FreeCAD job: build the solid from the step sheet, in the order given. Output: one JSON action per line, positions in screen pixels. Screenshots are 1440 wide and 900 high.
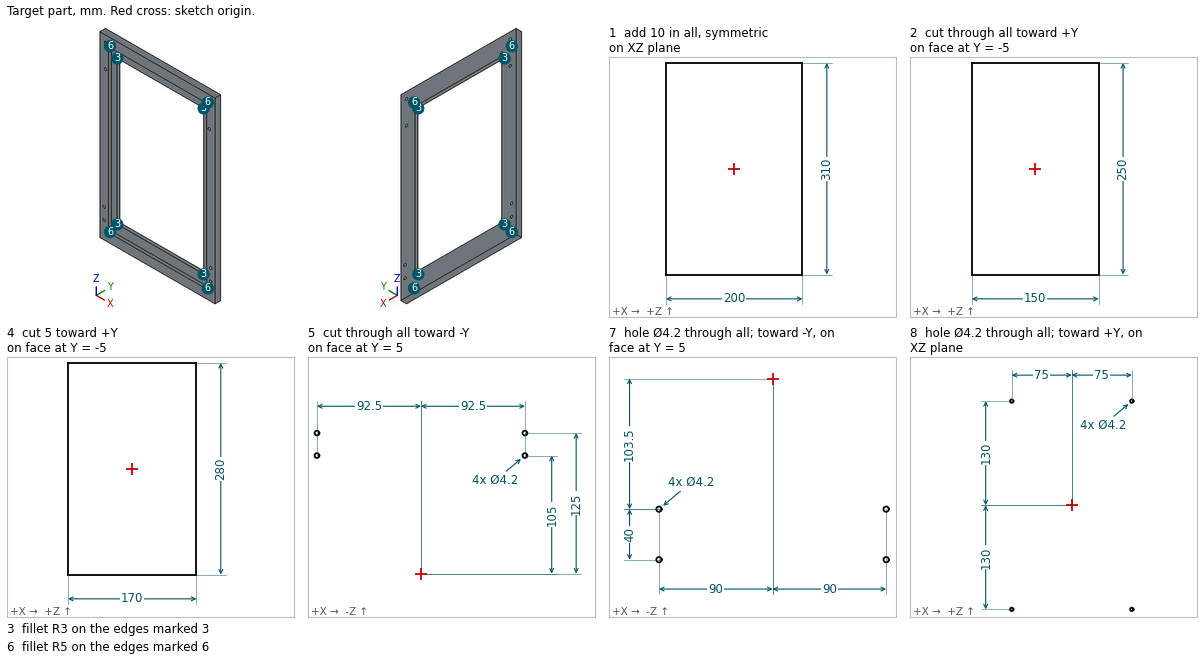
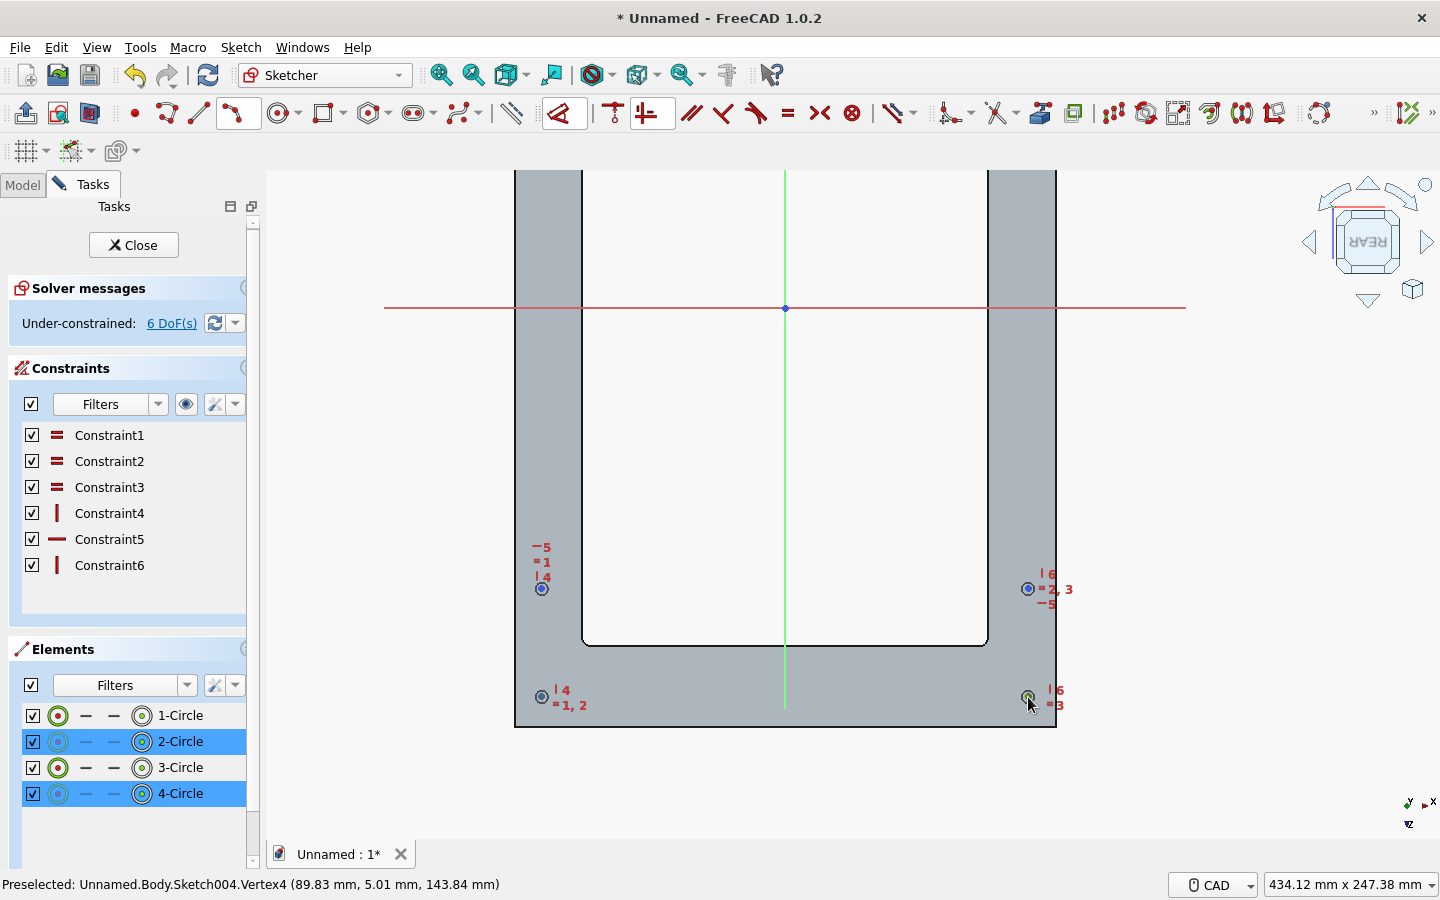
{"action": "left_click", "coordinate": [670, 114]}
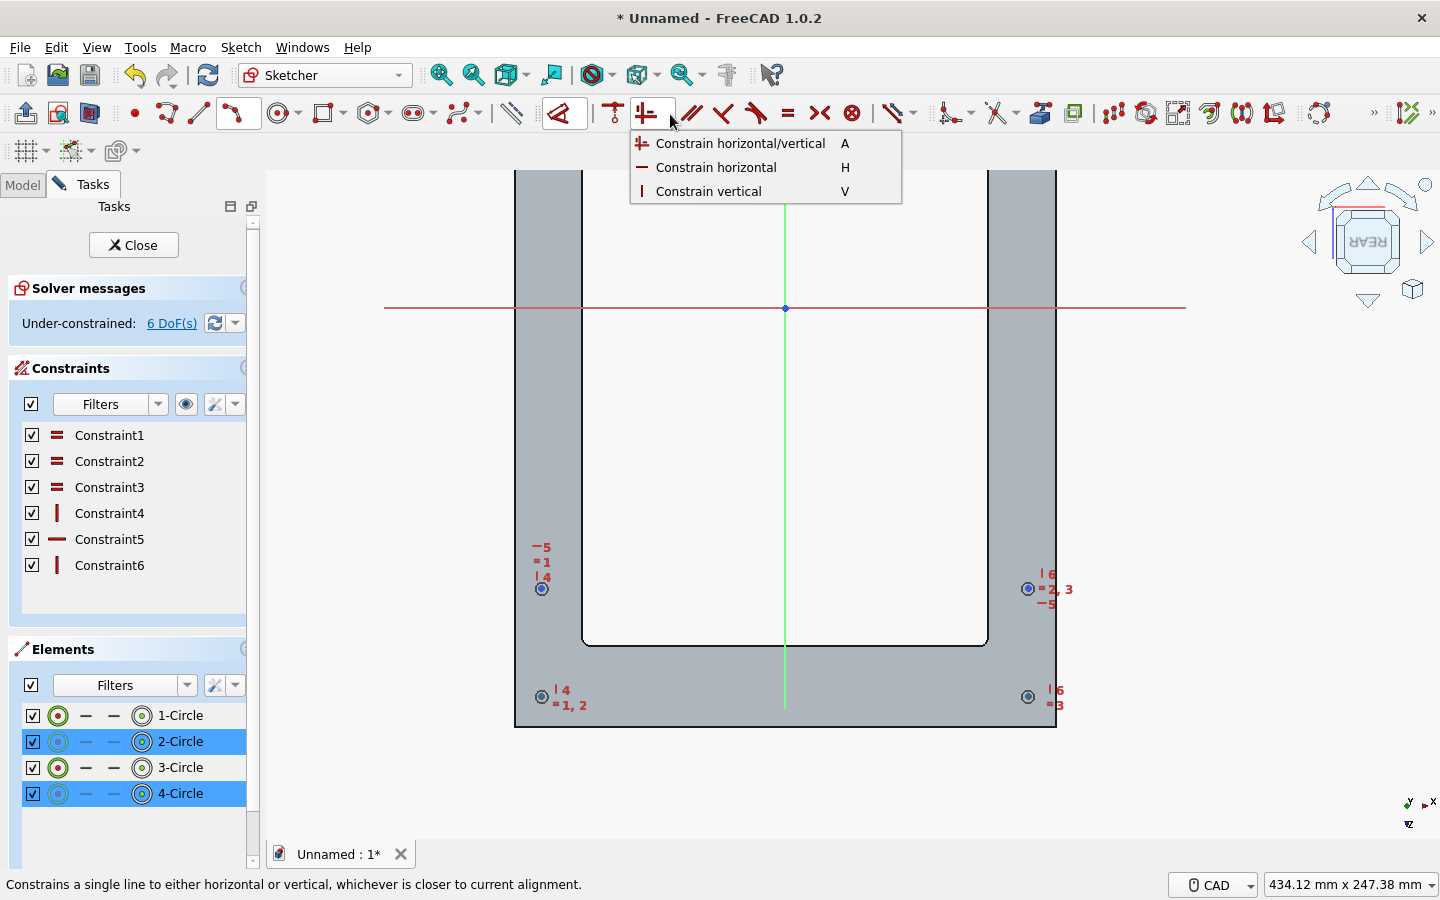
{"action": "left_click", "coordinate": [766, 167]}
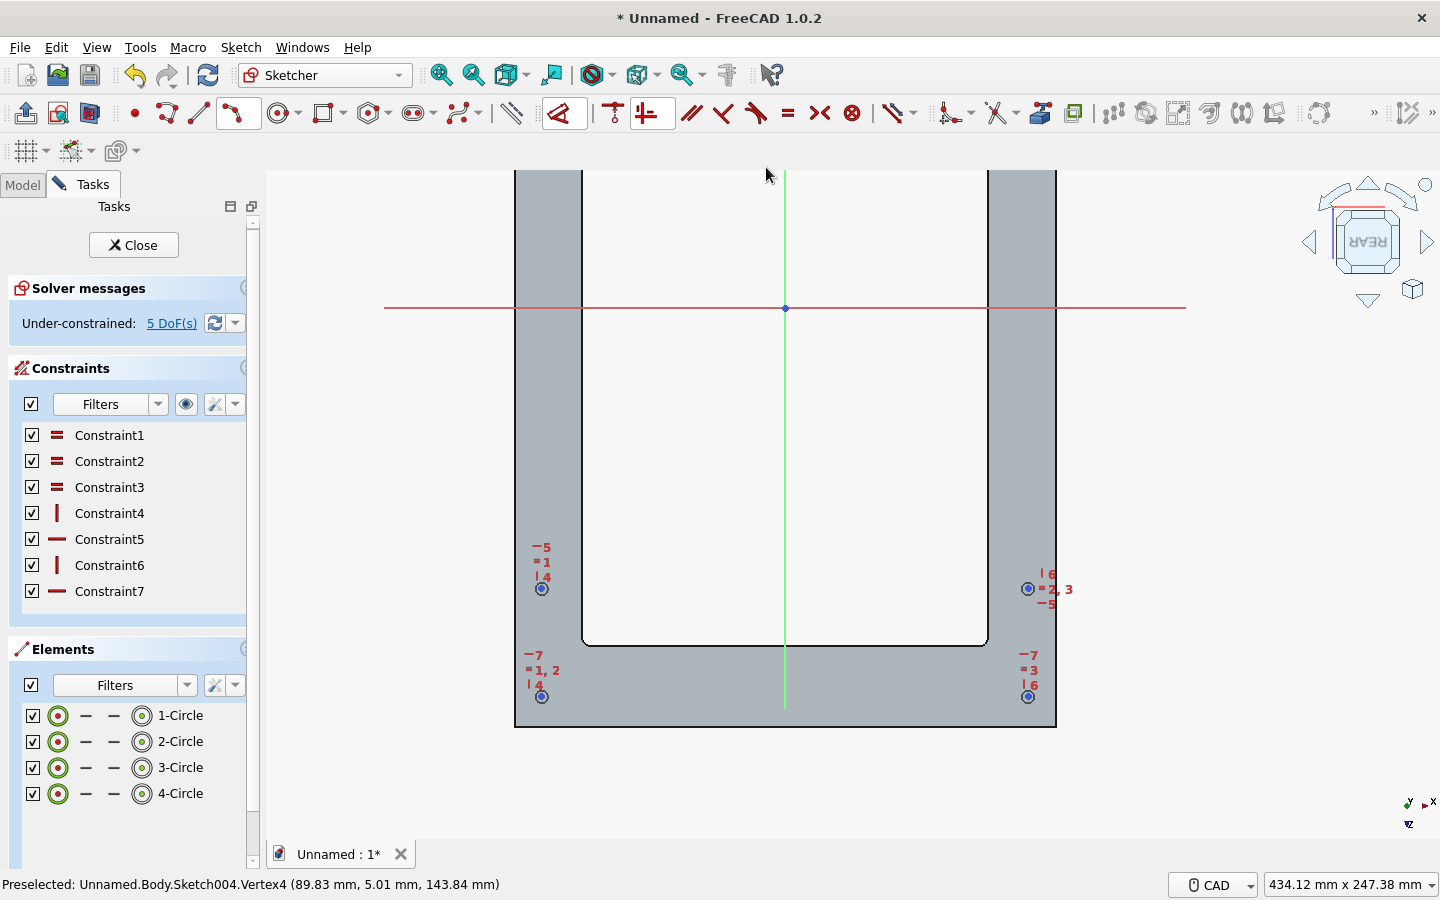
{"action": "scroll", "coordinate": [546, 585], "scroll_direction": "up", "scroll_amount": 7}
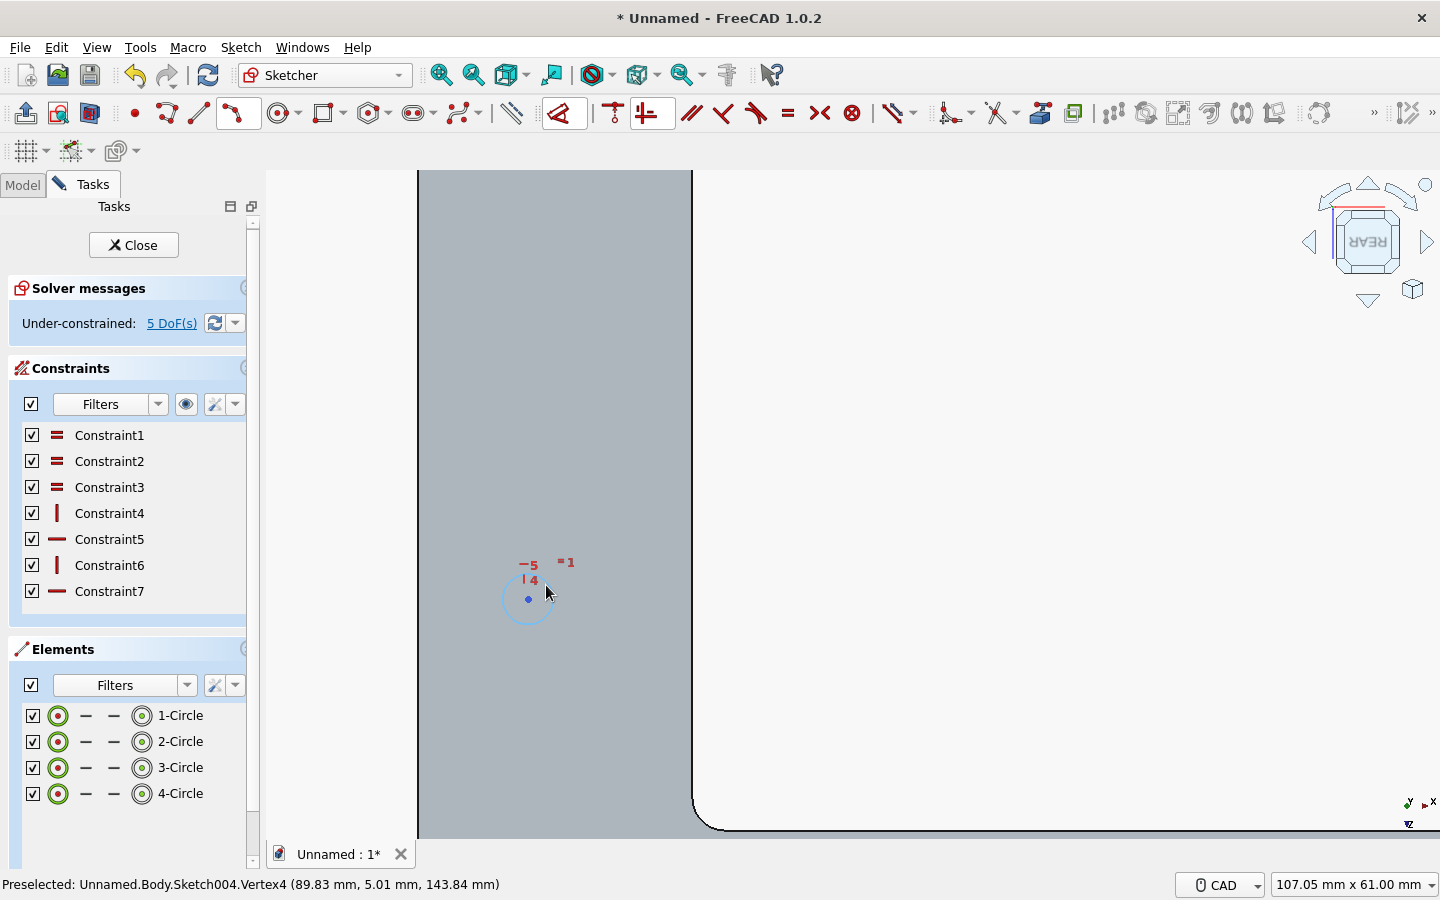
{"action": "left_click", "coordinate": [546, 581]}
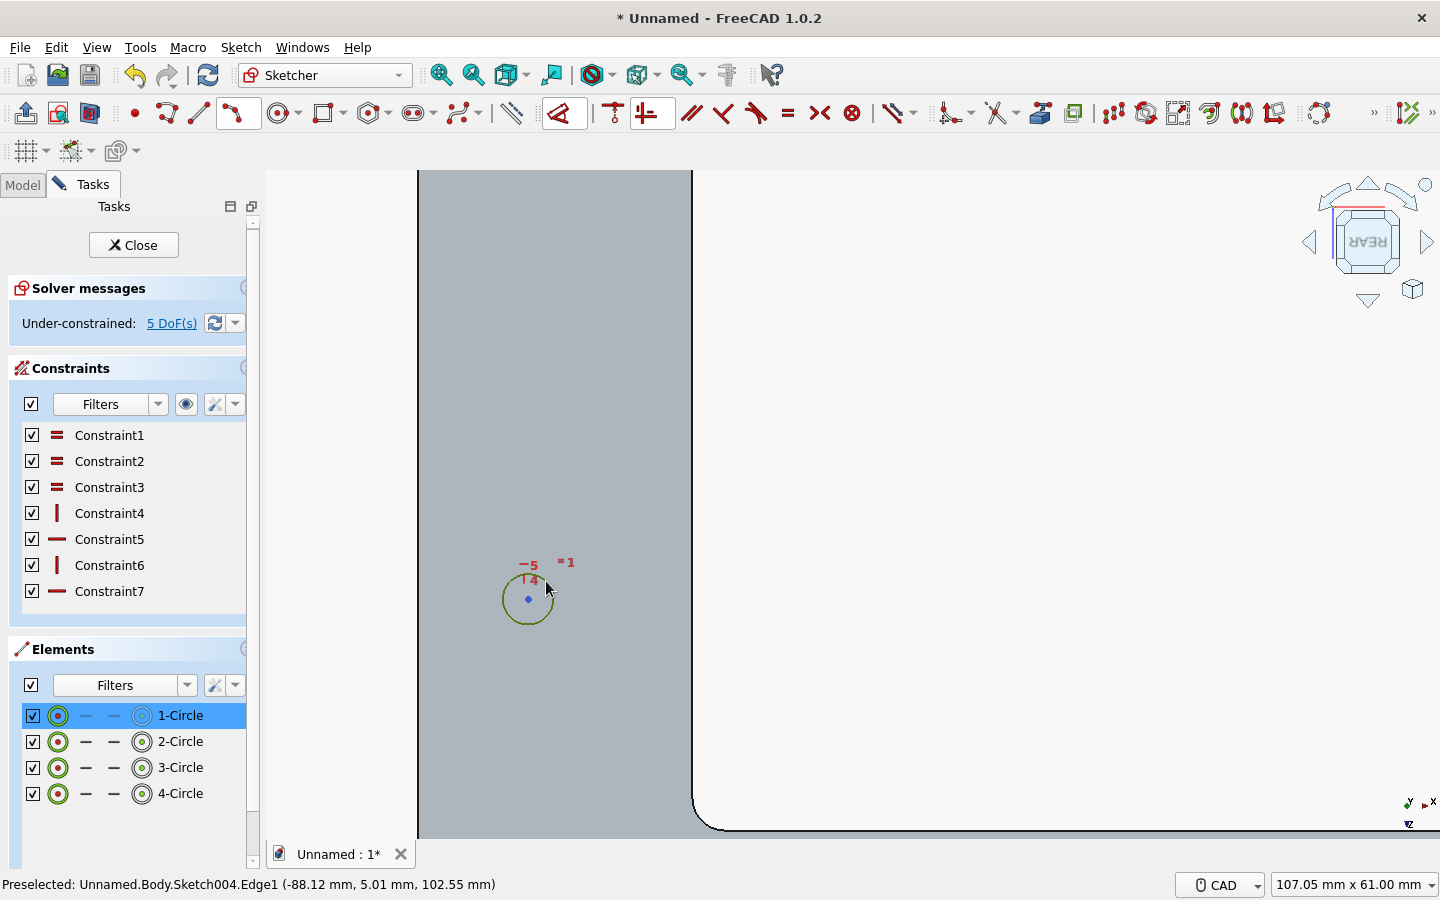
{"action": "key", "text": "k o"}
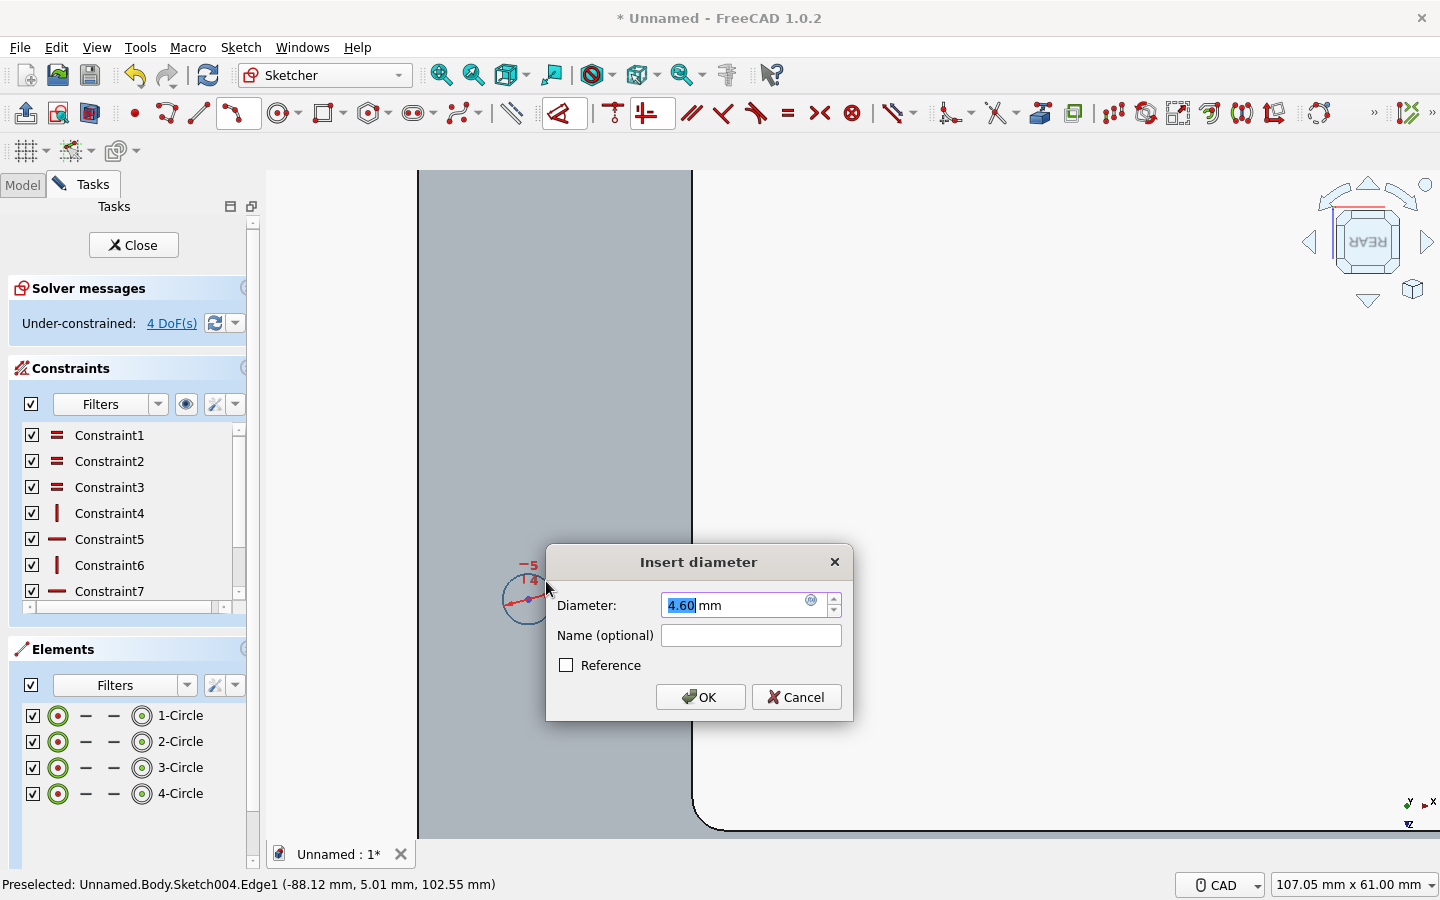
{"action": "type", "text": "4.2"}
{"action": "key", "text": "Return"}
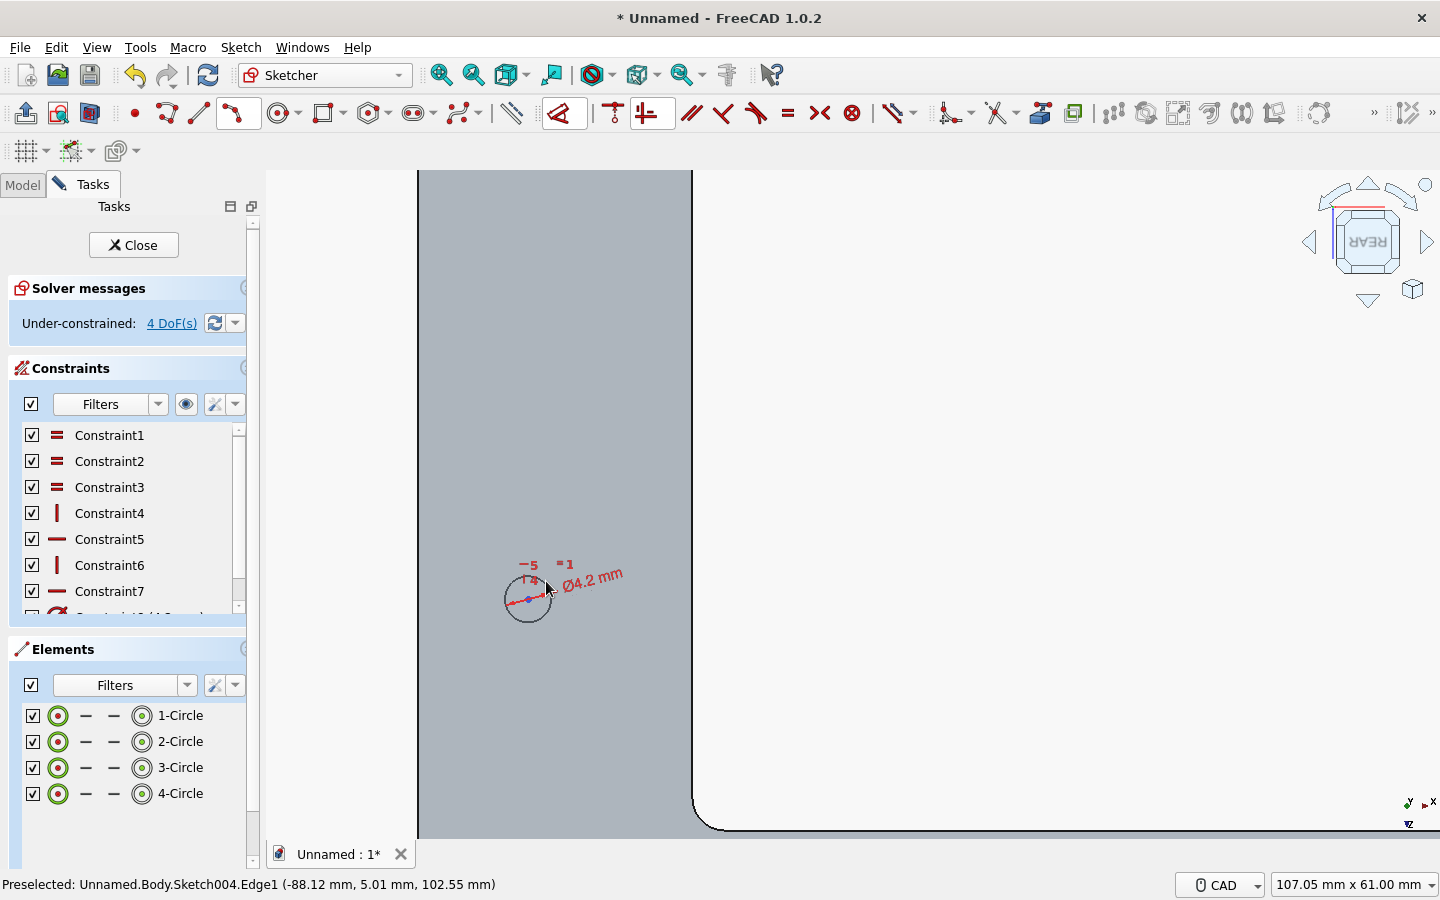
{"action": "scroll", "coordinate": [545, 585], "scroll_direction": "down", "scroll_amount": 7}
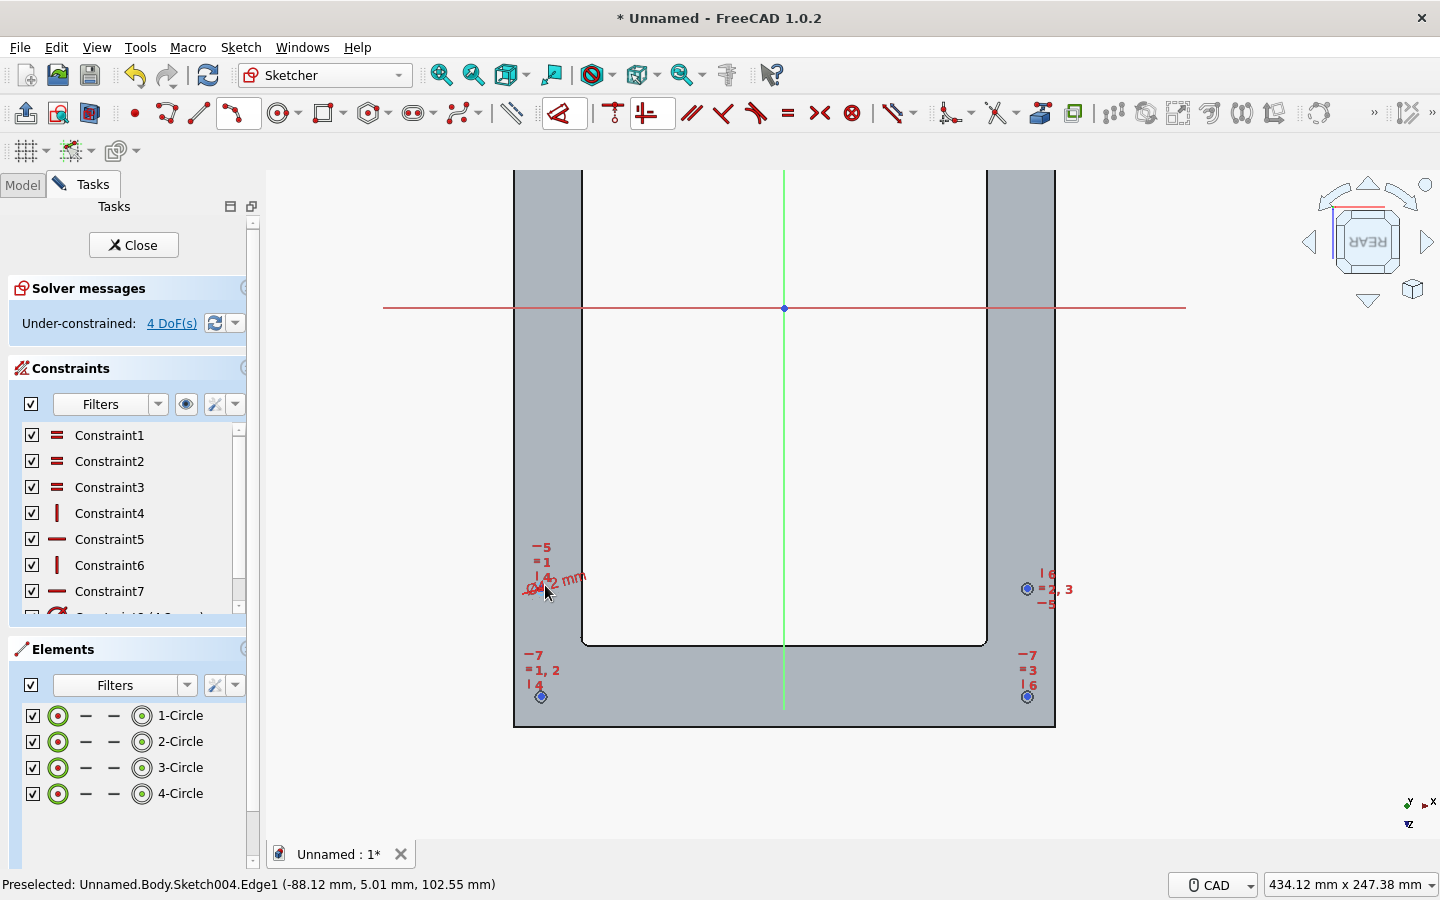
{"action": "left_click", "coordinate": [541, 589]}